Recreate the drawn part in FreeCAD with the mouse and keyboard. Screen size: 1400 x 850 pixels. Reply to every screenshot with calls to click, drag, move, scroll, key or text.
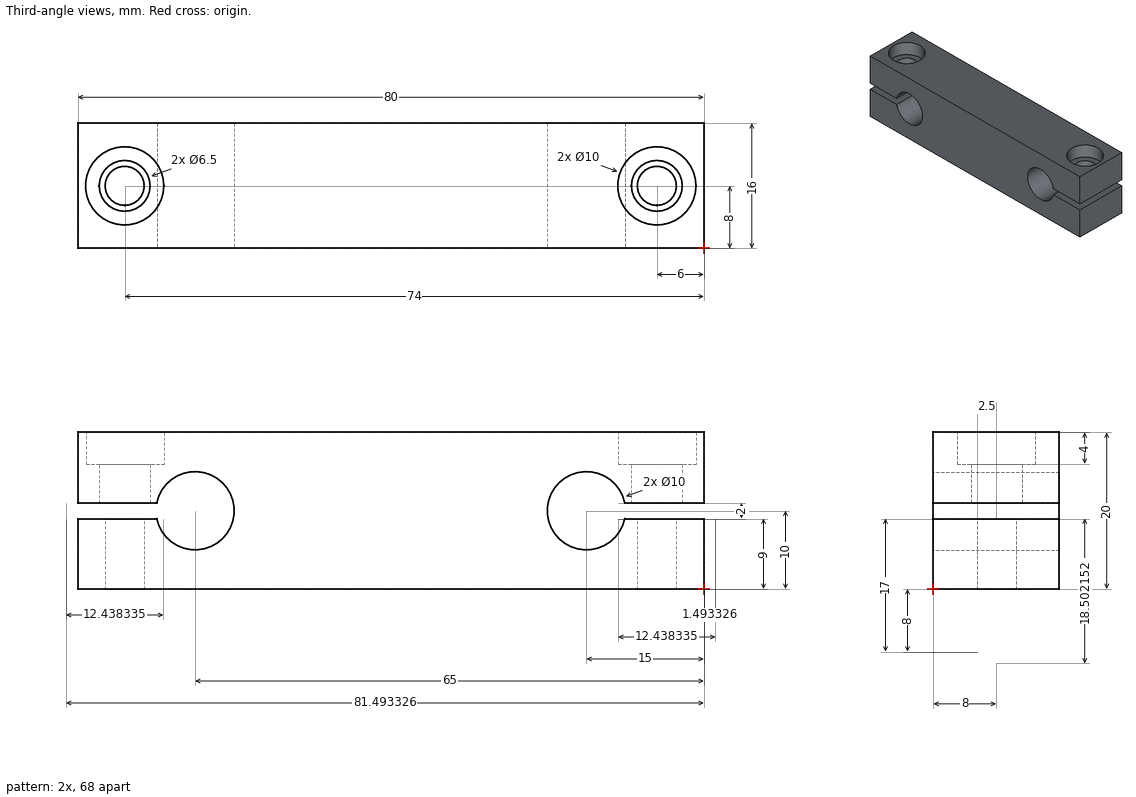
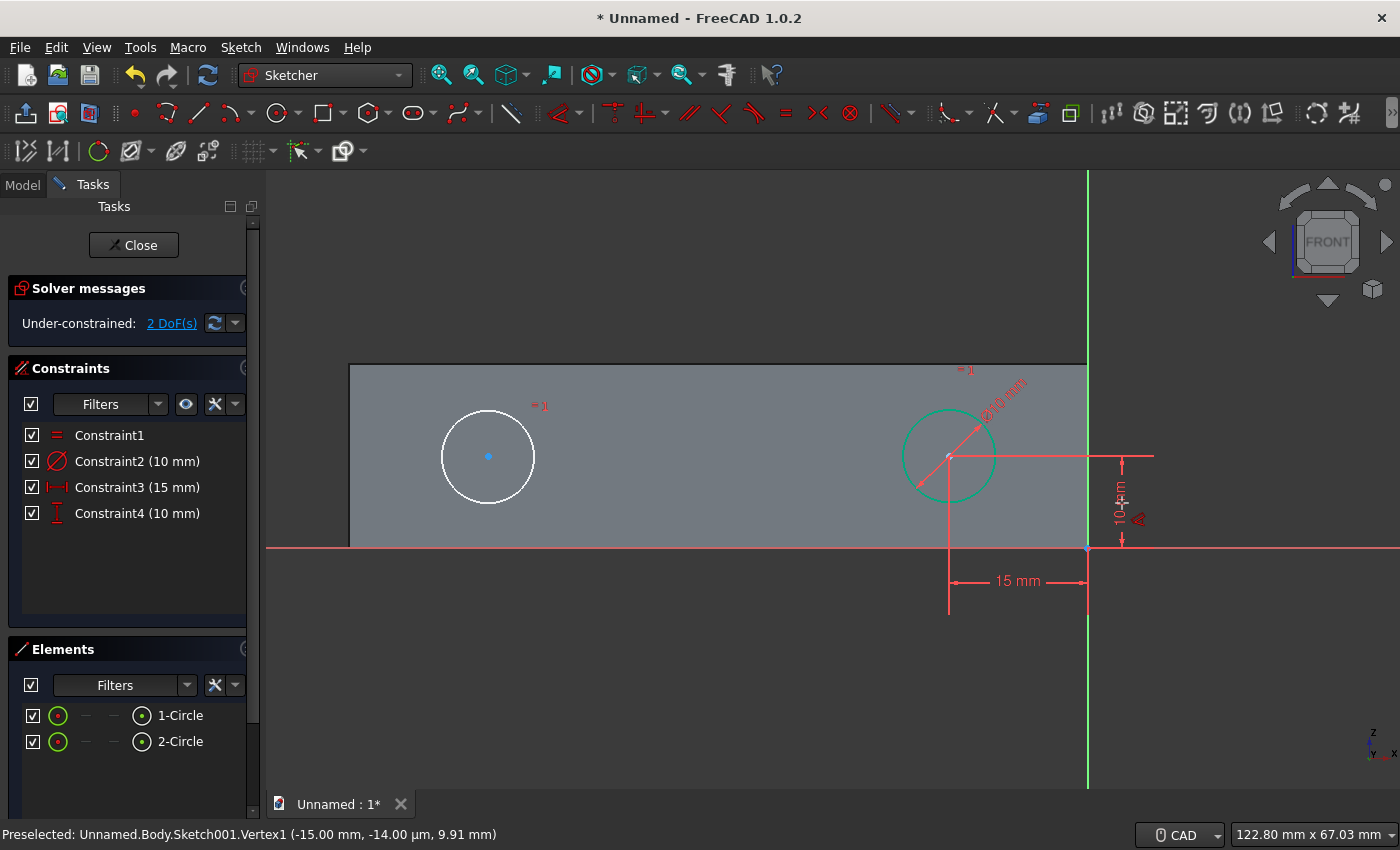
click(488, 457)
click(788, 582)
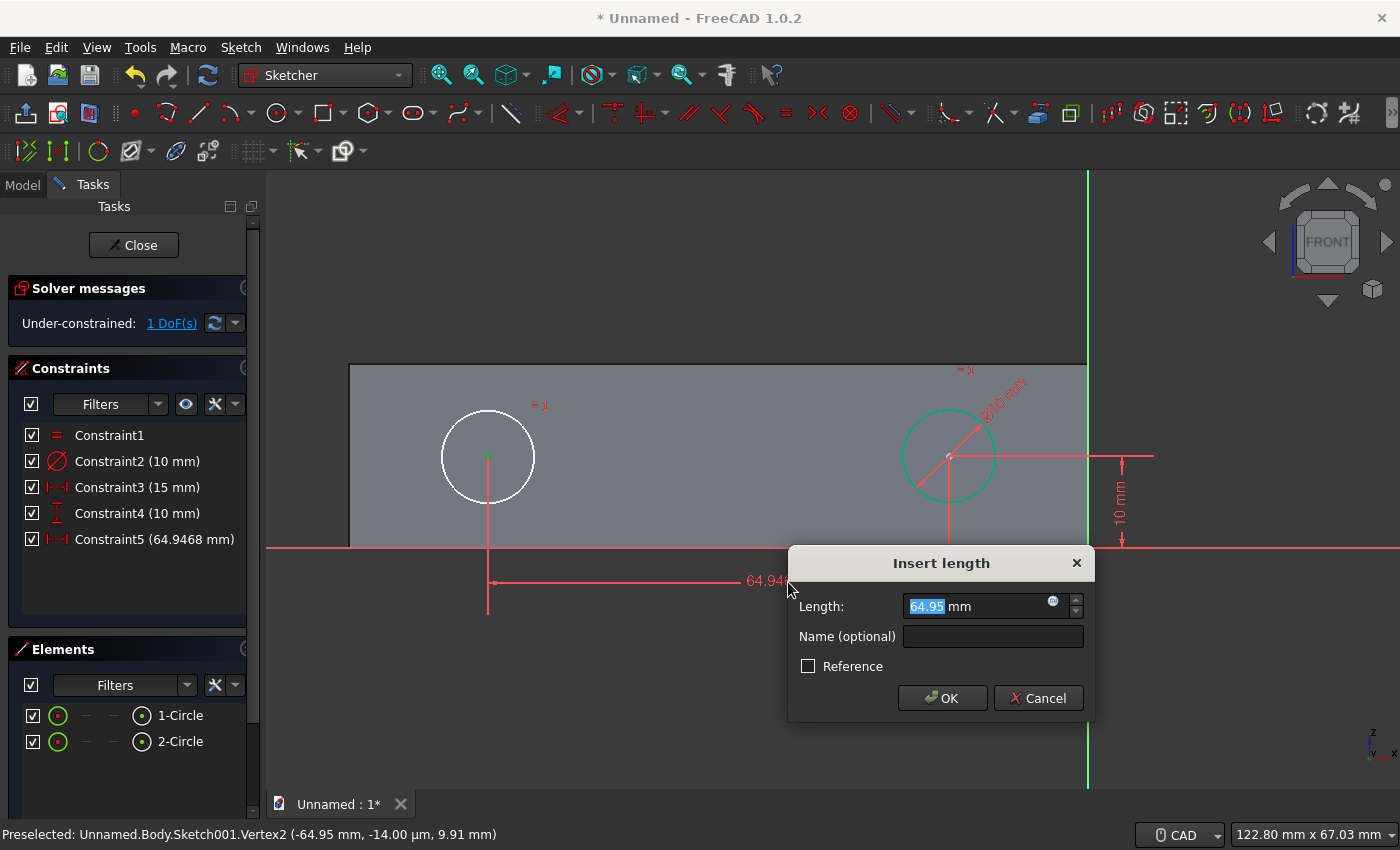
text(65)
key(Return)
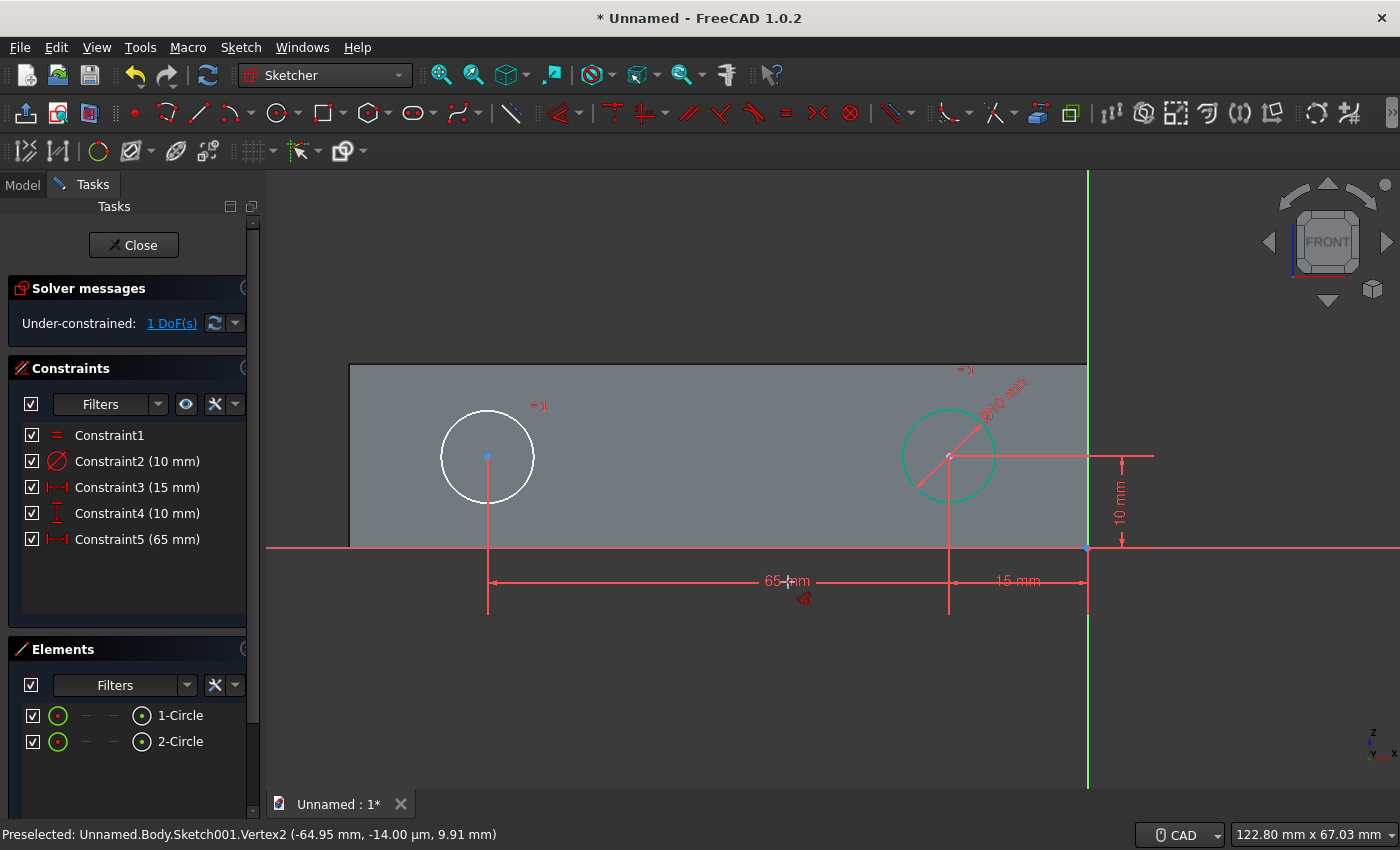
click(488, 457)
click(1122, 482)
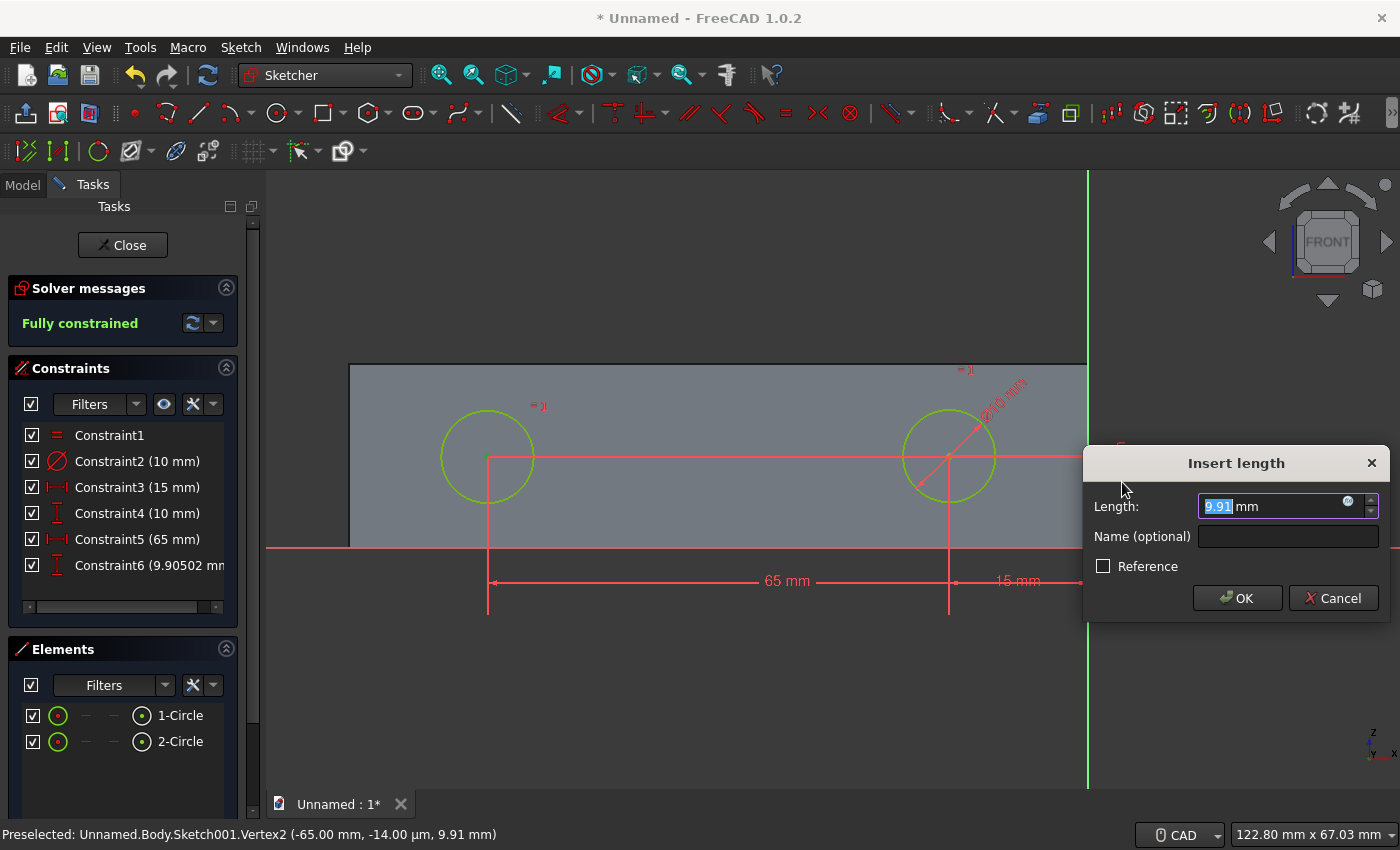
text(10)
key(Return)
key(Escape)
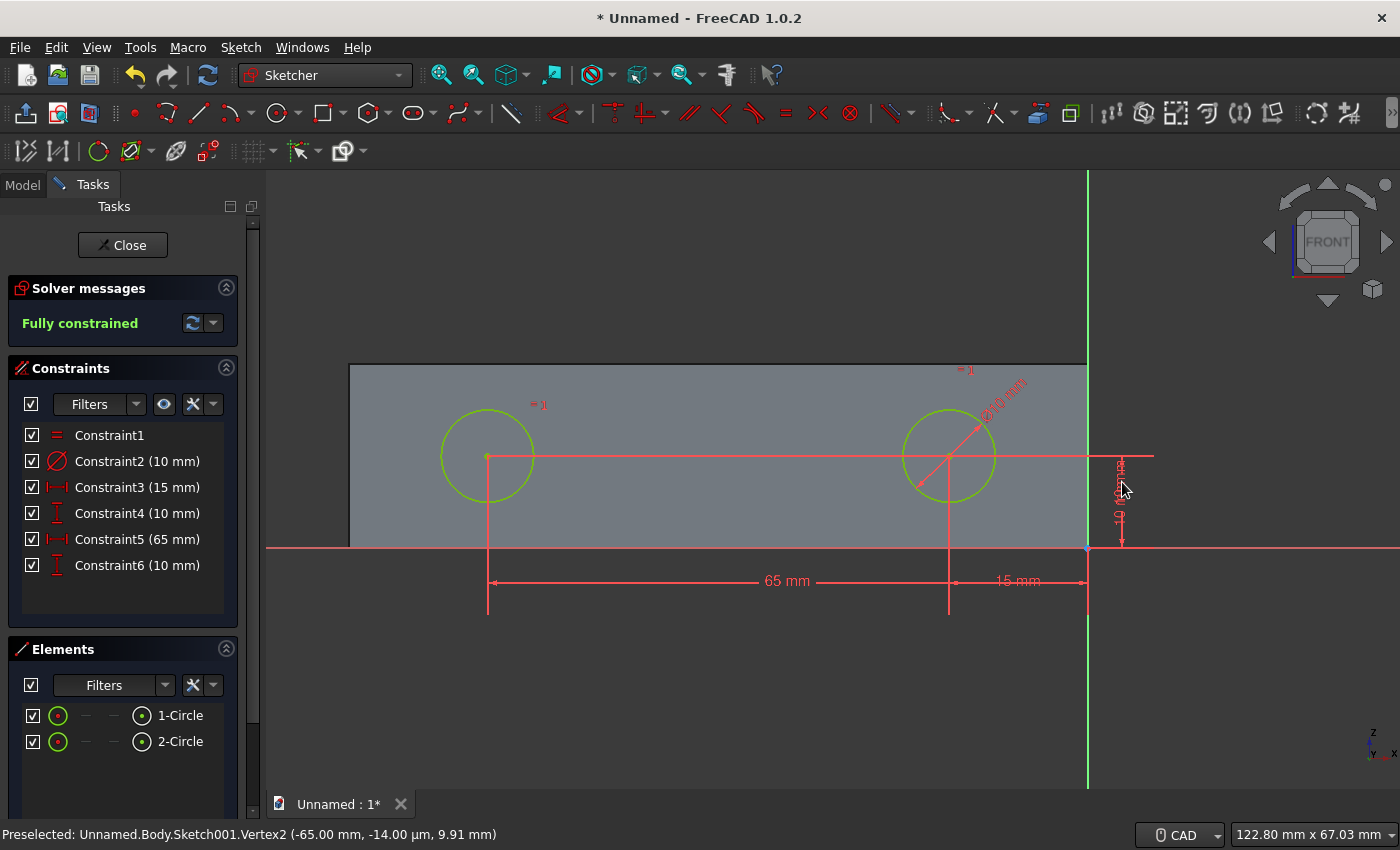
click(123, 245)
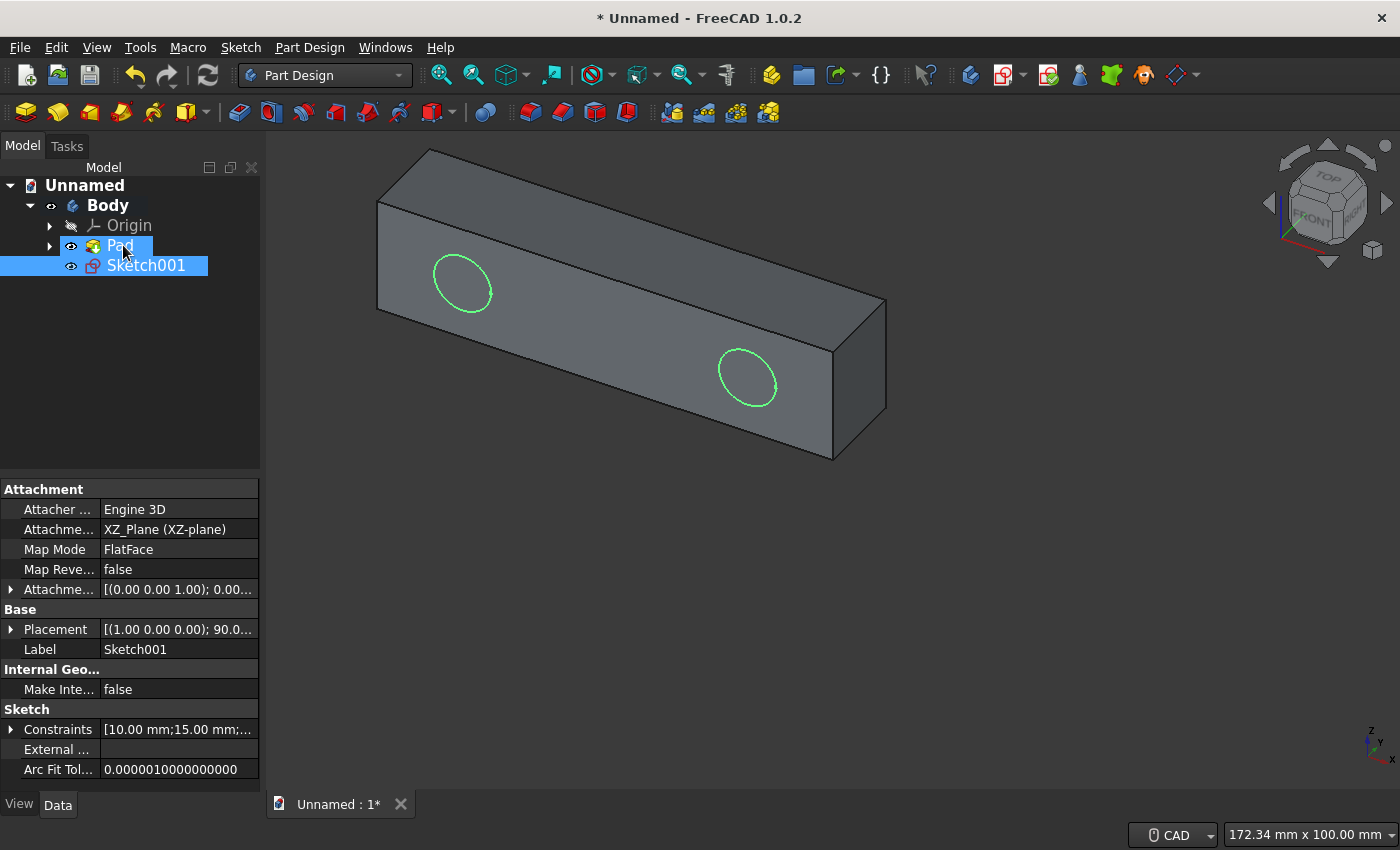
click(240, 112)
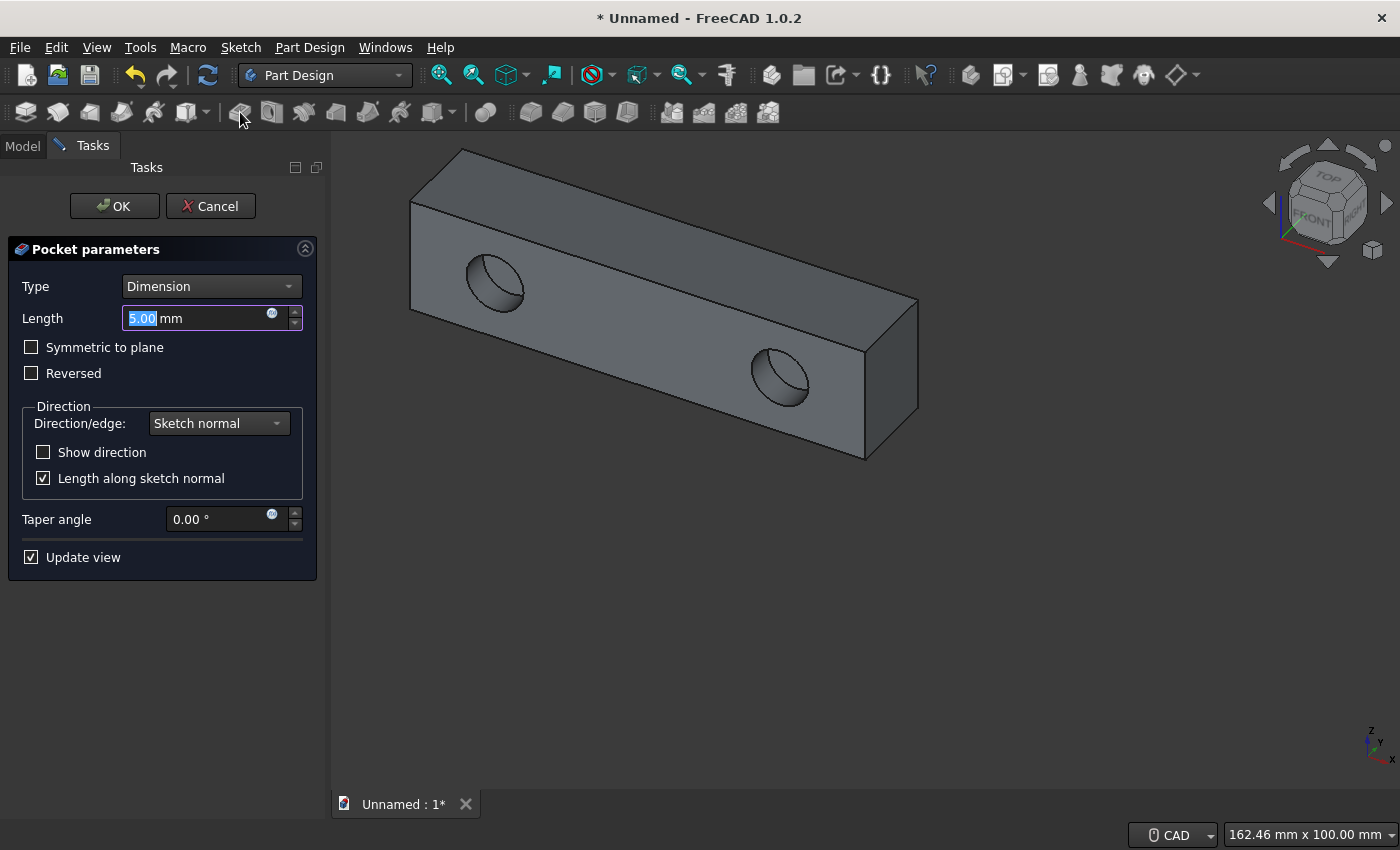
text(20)
key(Tab)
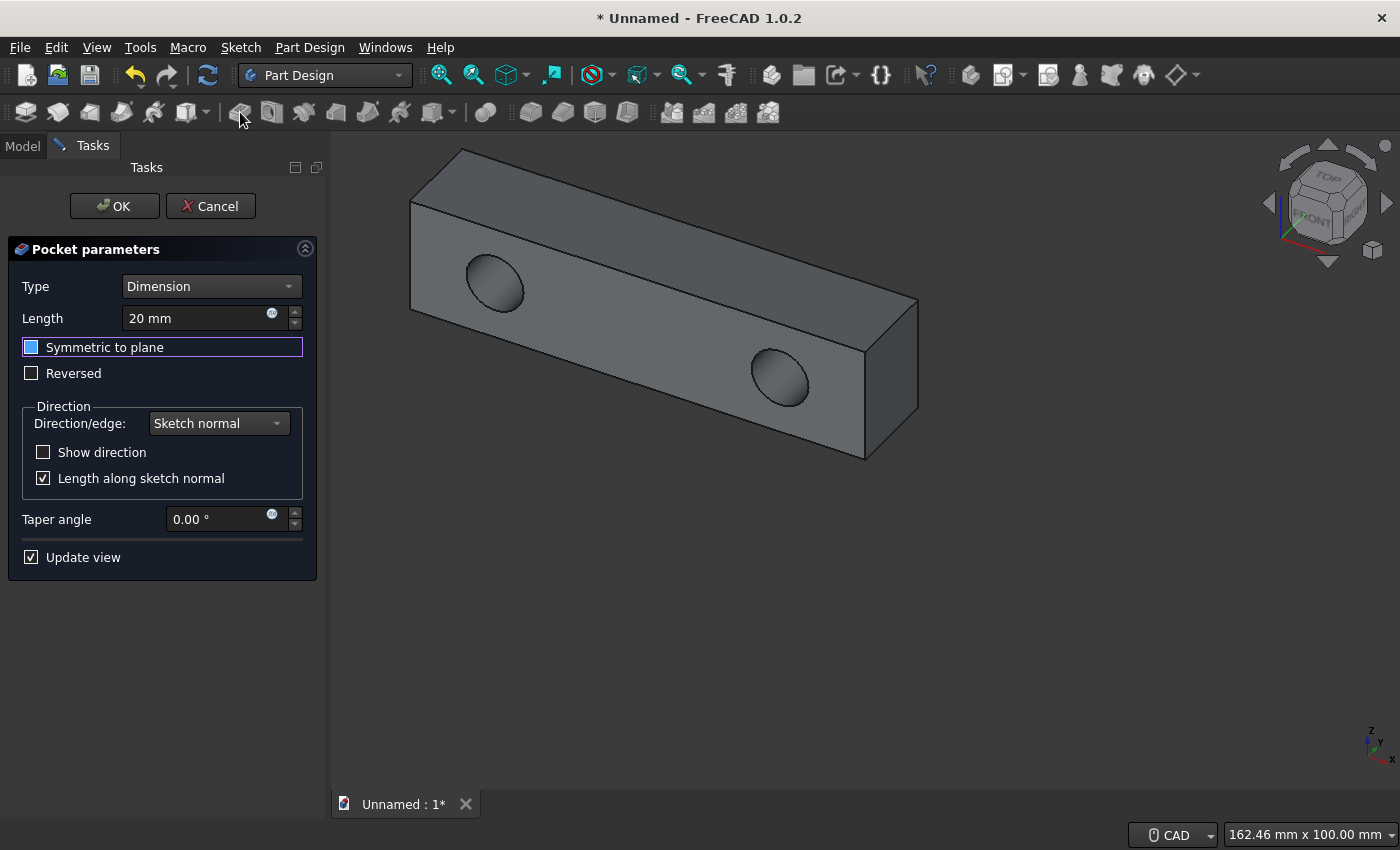
click(115, 206)